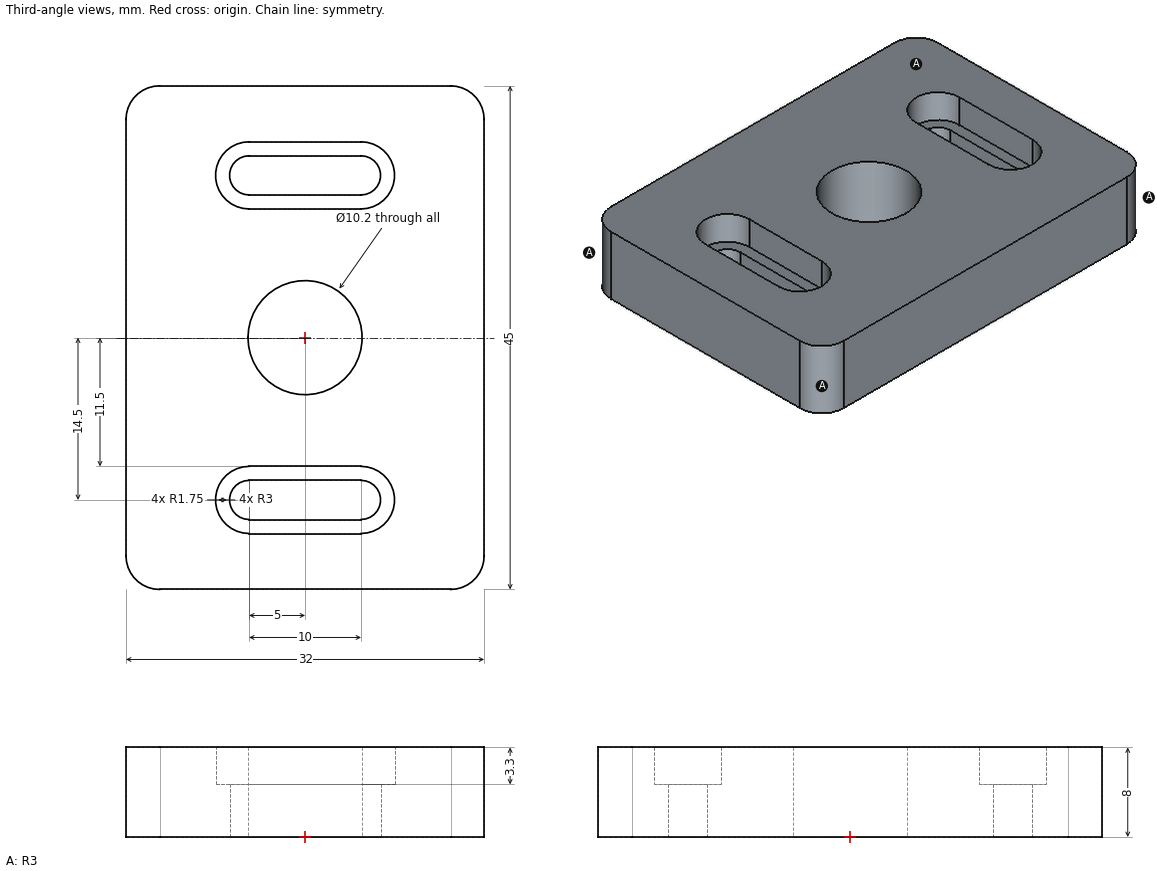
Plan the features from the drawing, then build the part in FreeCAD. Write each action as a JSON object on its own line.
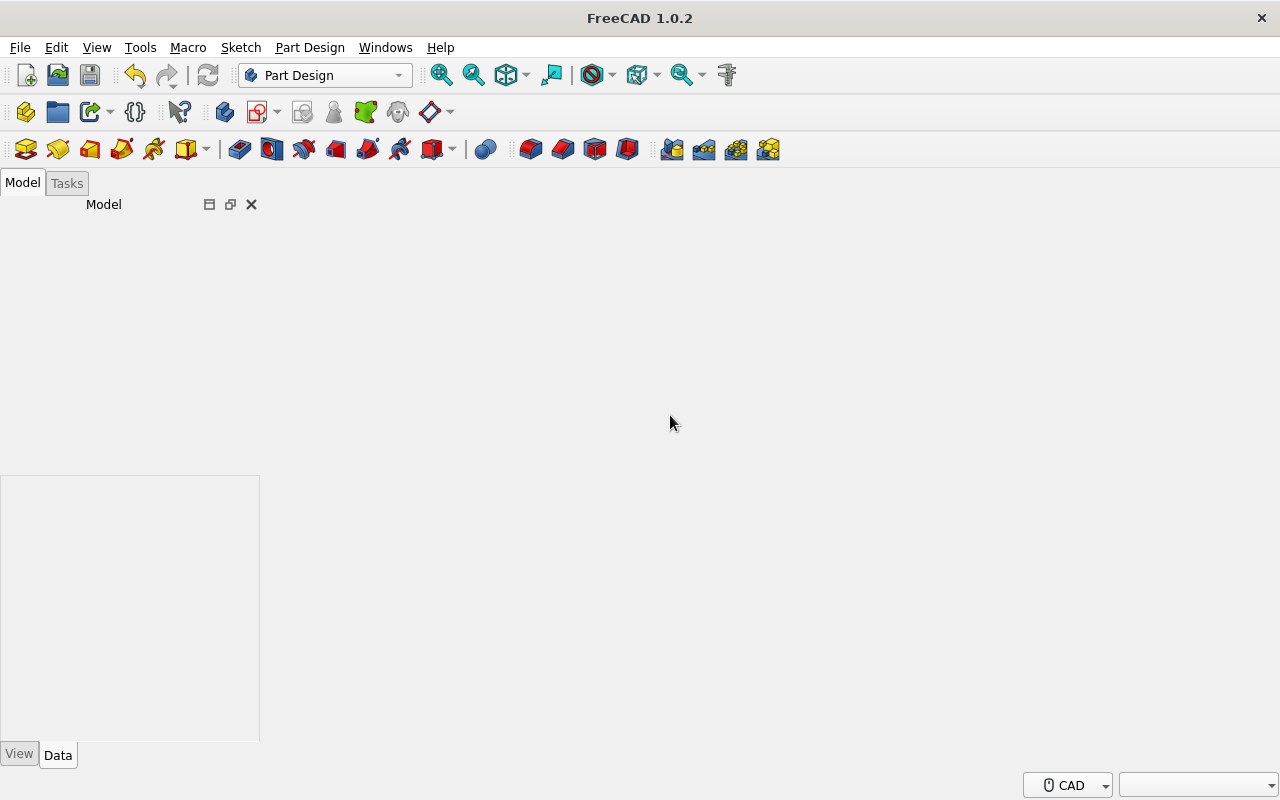
{"action": "left_click", "coordinate": [26, 76]}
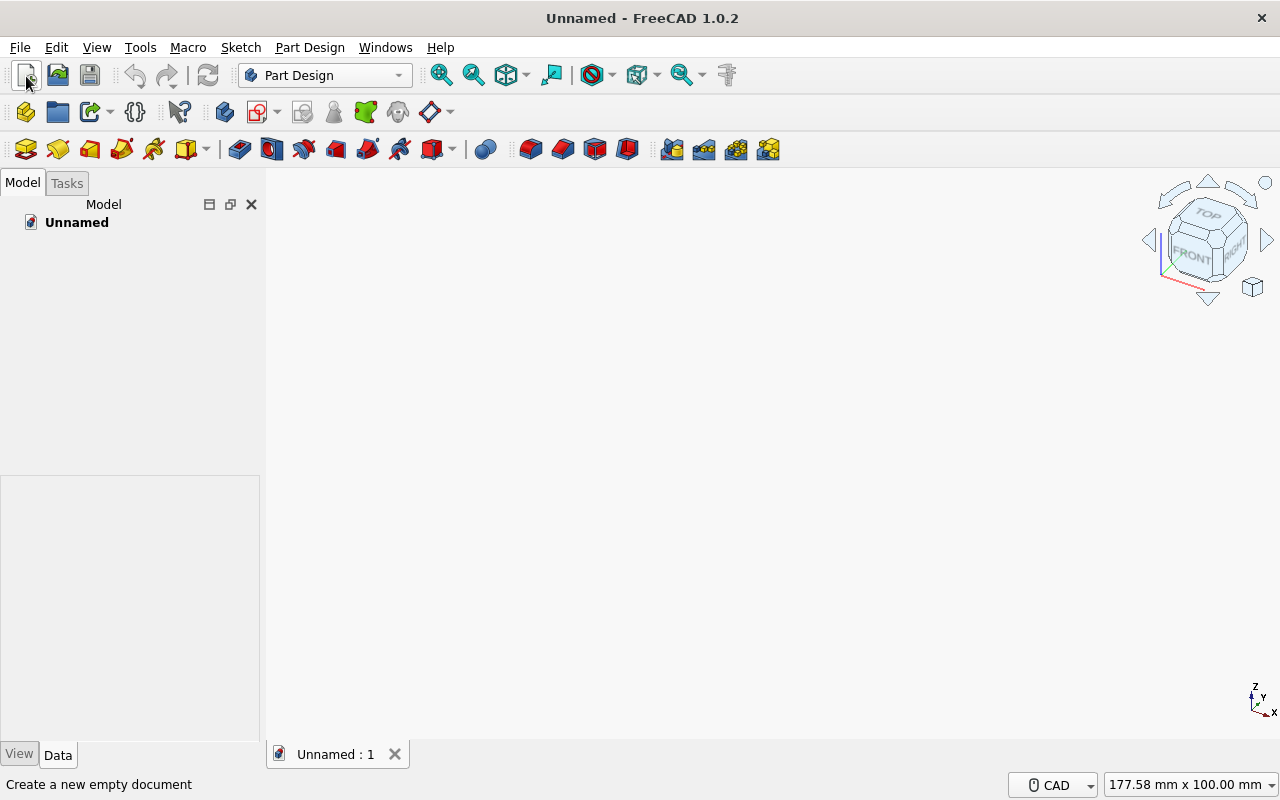
{"action": "left_click", "coordinate": [258, 112]}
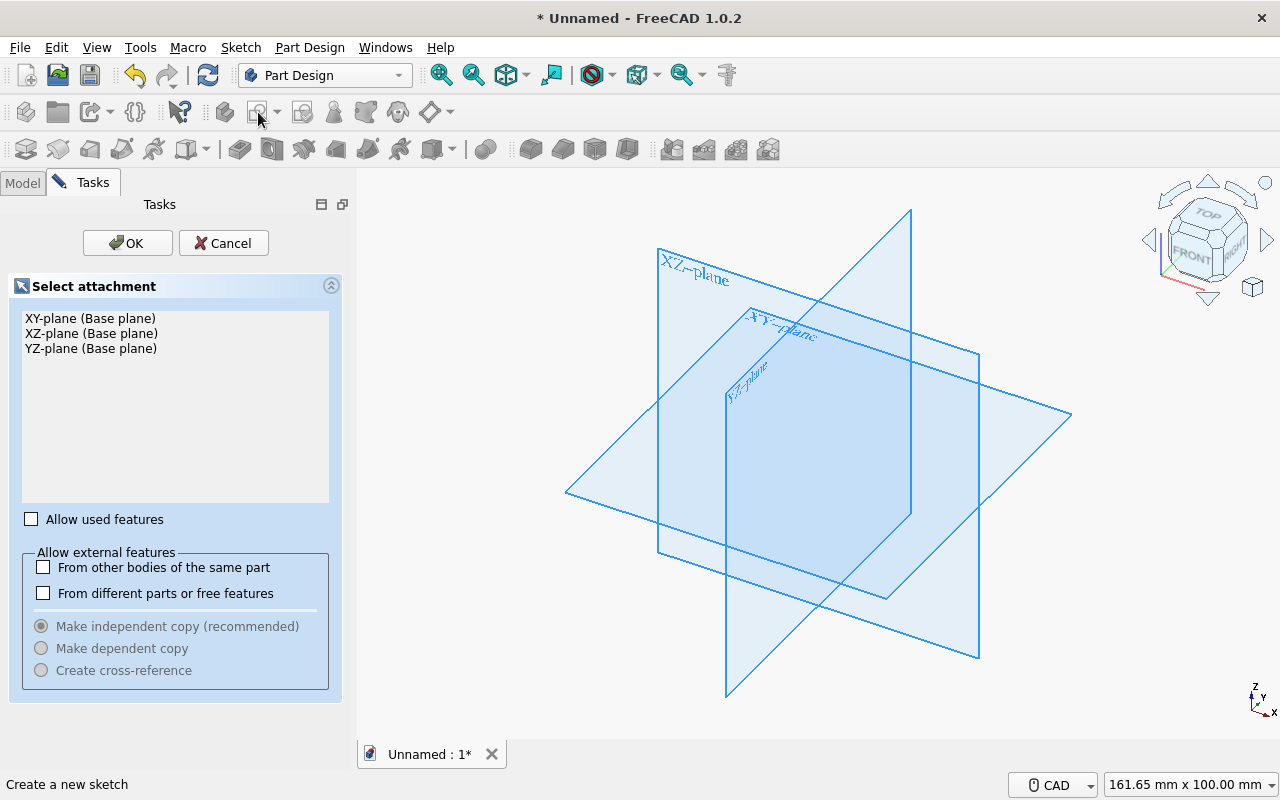
{"action": "left_click", "coordinate": [82, 318]}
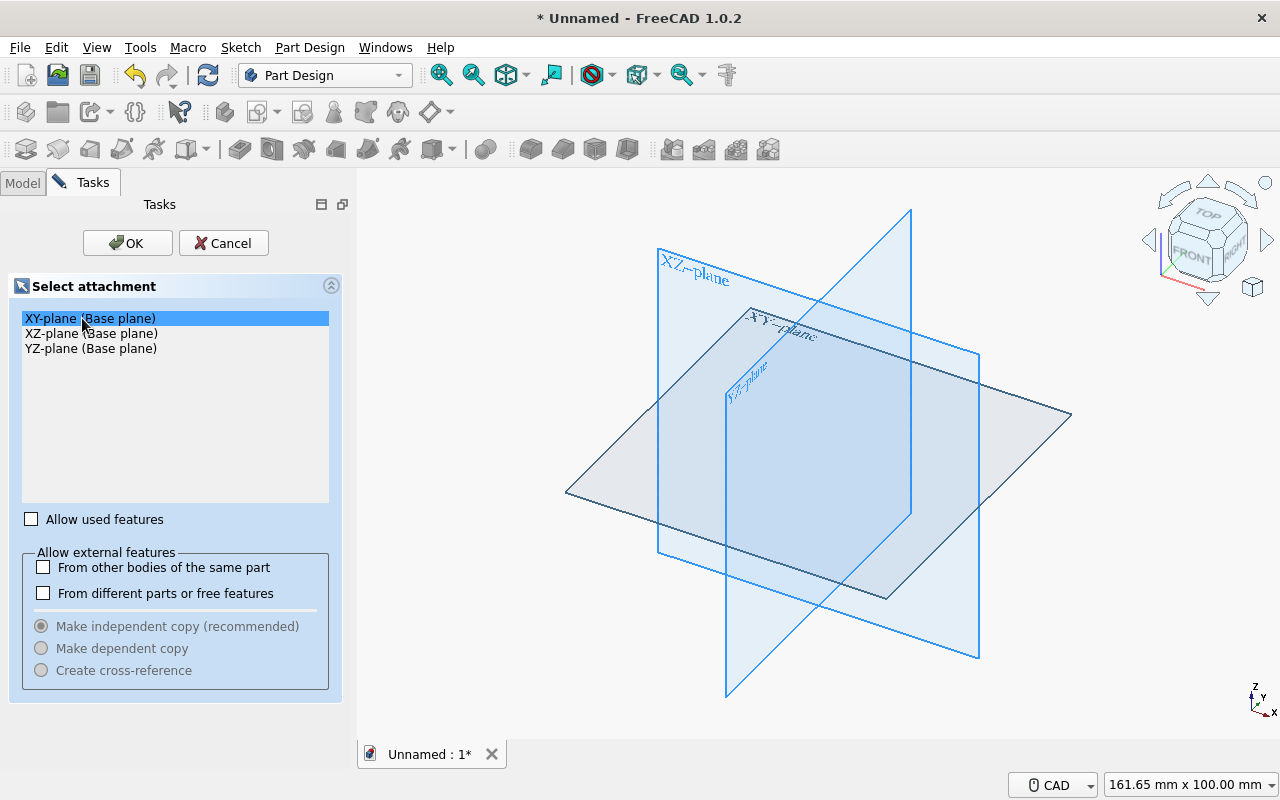
{"action": "left_click", "coordinate": [128, 243]}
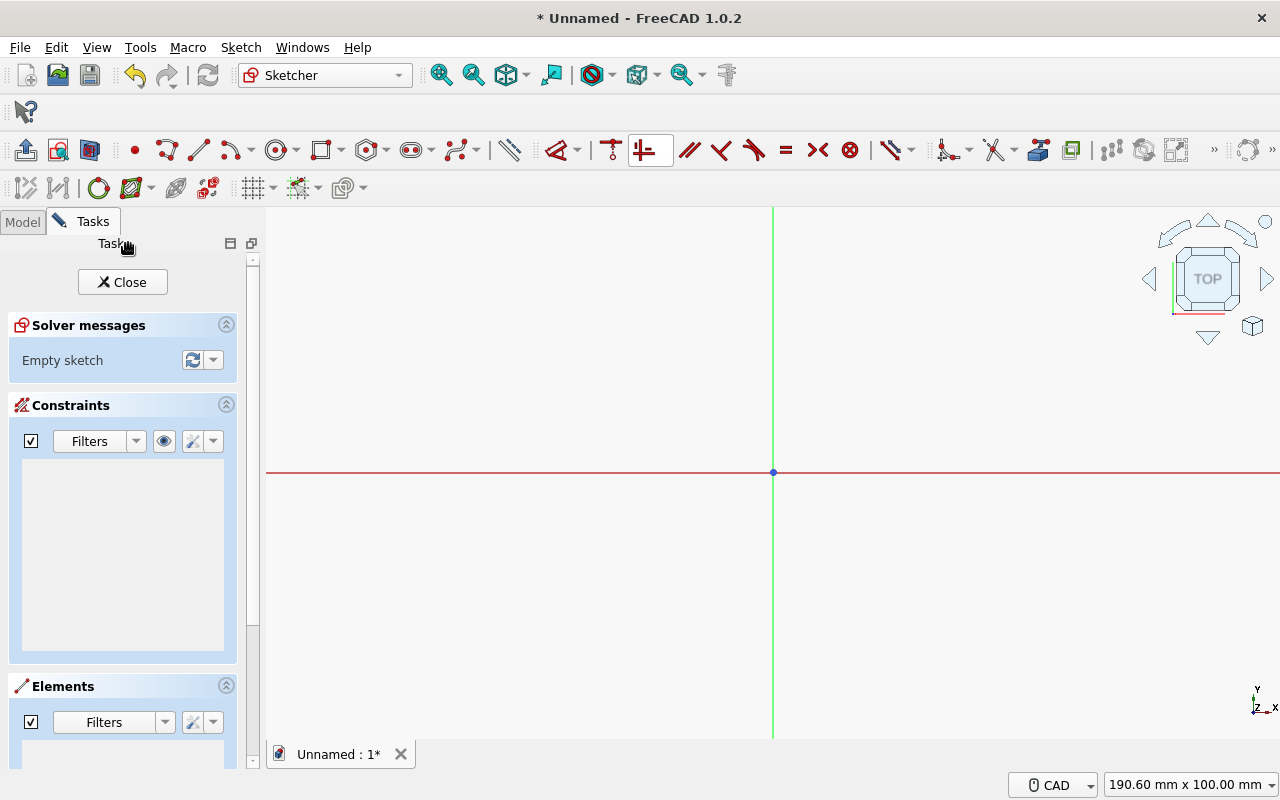
{"action": "scroll", "coordinate": [912, 473], "scroll_direction": "up", "scroll_amount": 2}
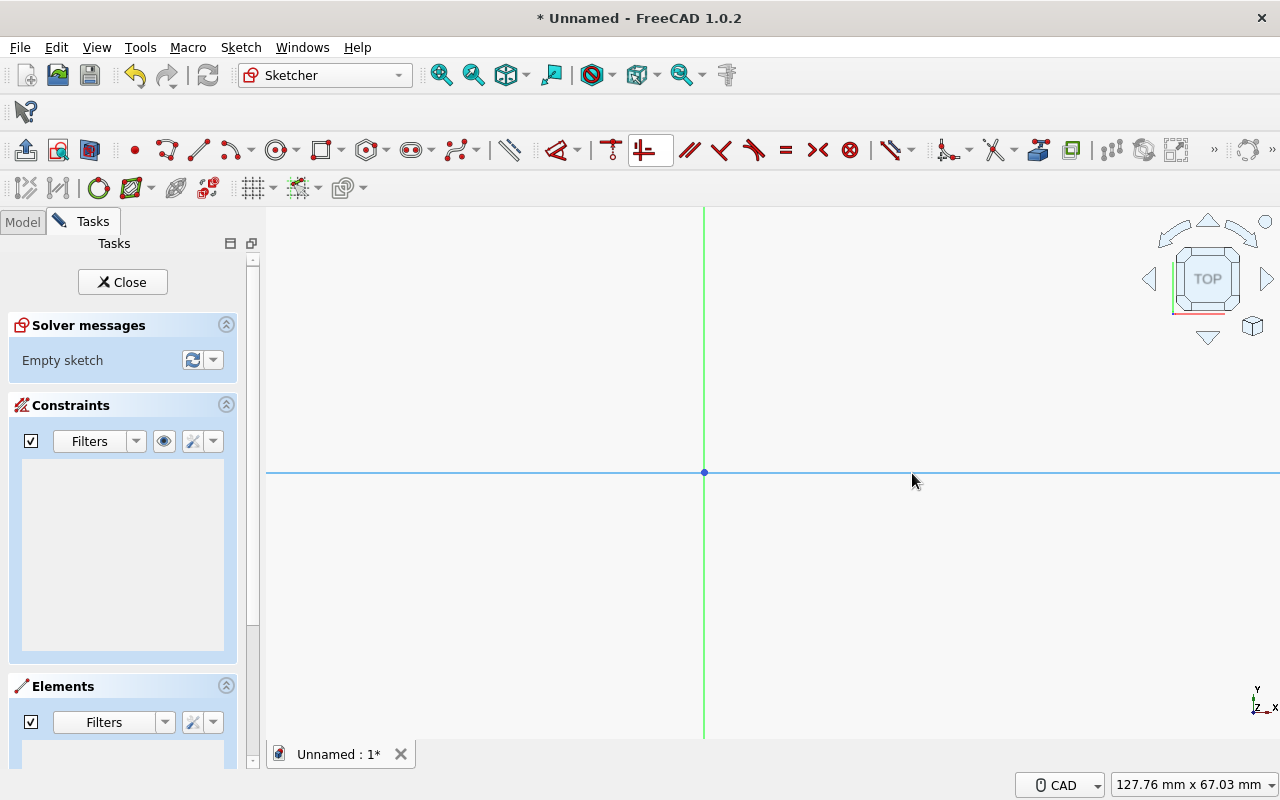
{"action": "left_click", "coordinate": [344, 150]}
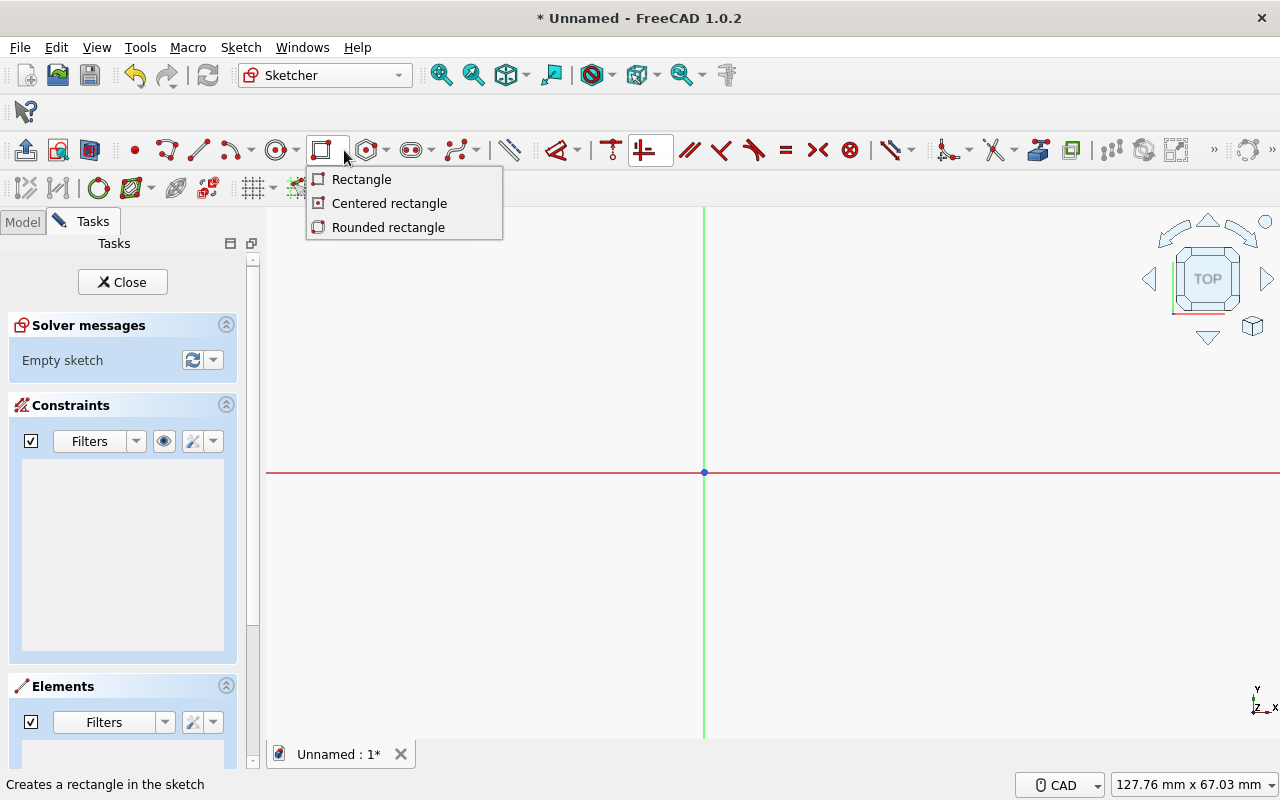
{"action": "left_click", "coordinate": [404, 203]}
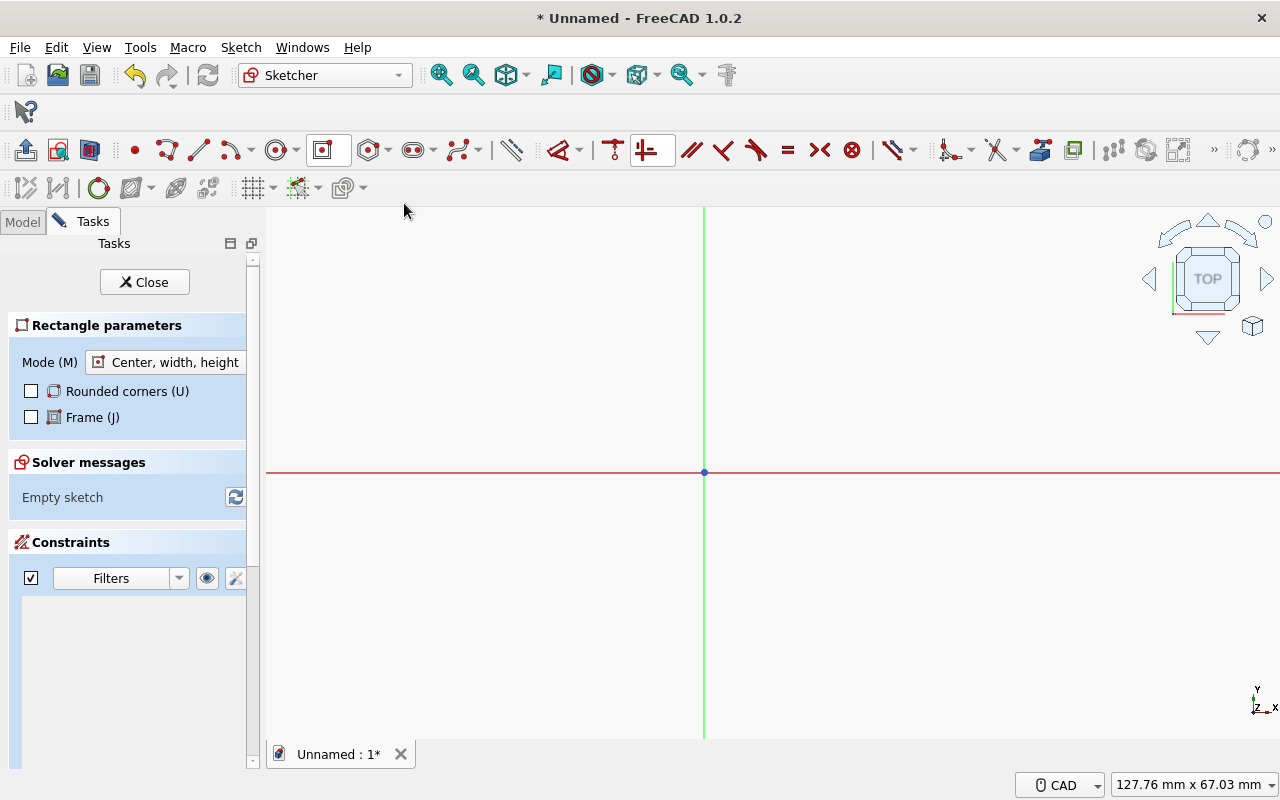
{"action": "left_click", "coordinate": [704, 473]}
{"action": "mouse_move", "coordinate": [831, 294]}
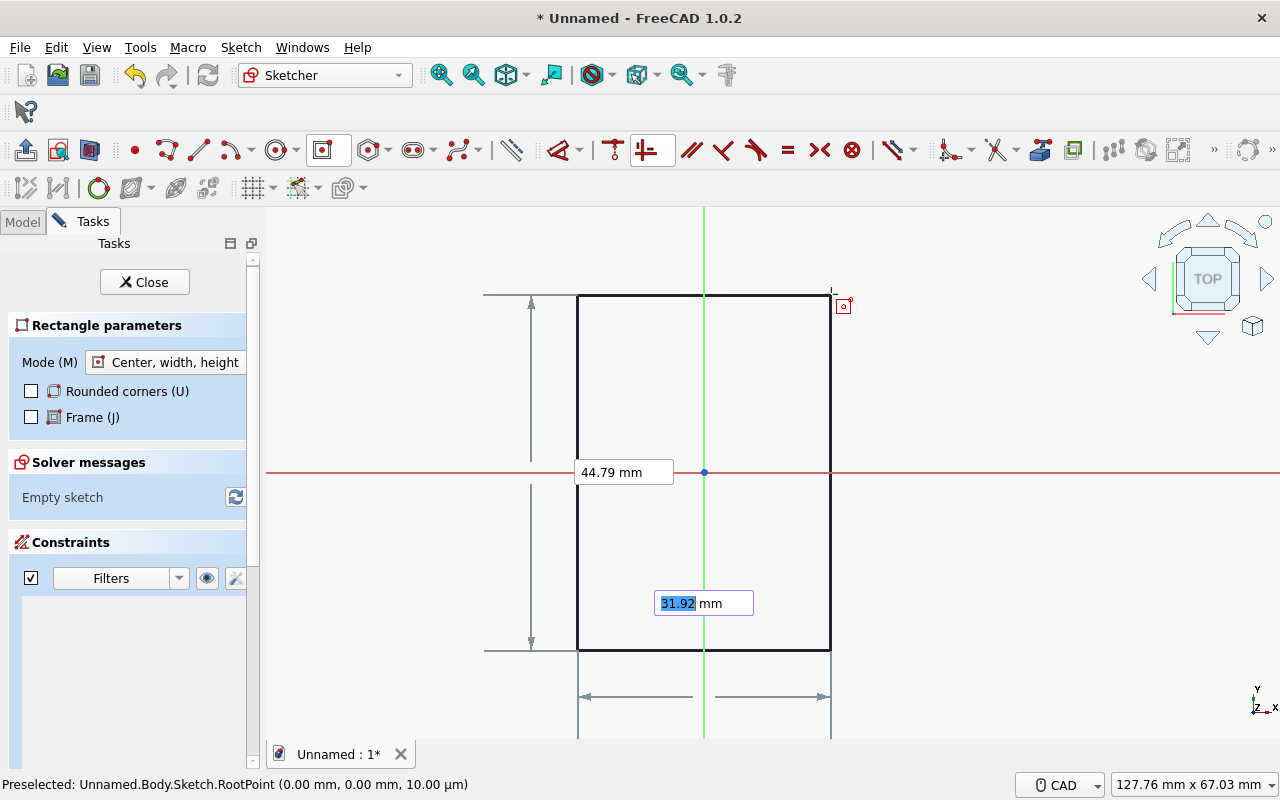
{"action": "type", "text": "32"}
{"action": "key", "text": "Tab"}
{"action": "type", "text": "45"}
{"action": "key", "text": "Return"}
{"action": "key", "text": "Escape"}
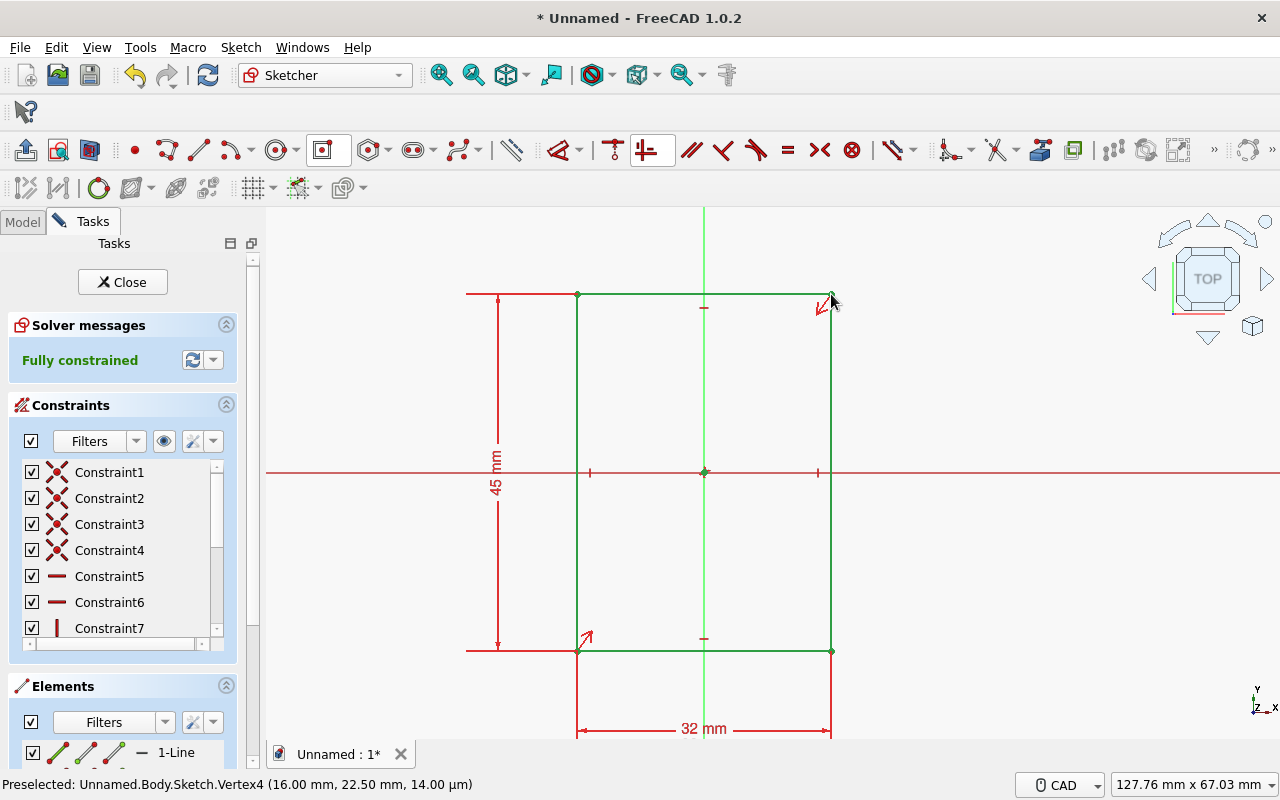
{"action": "left_click", "coordinate": [123, 282]}